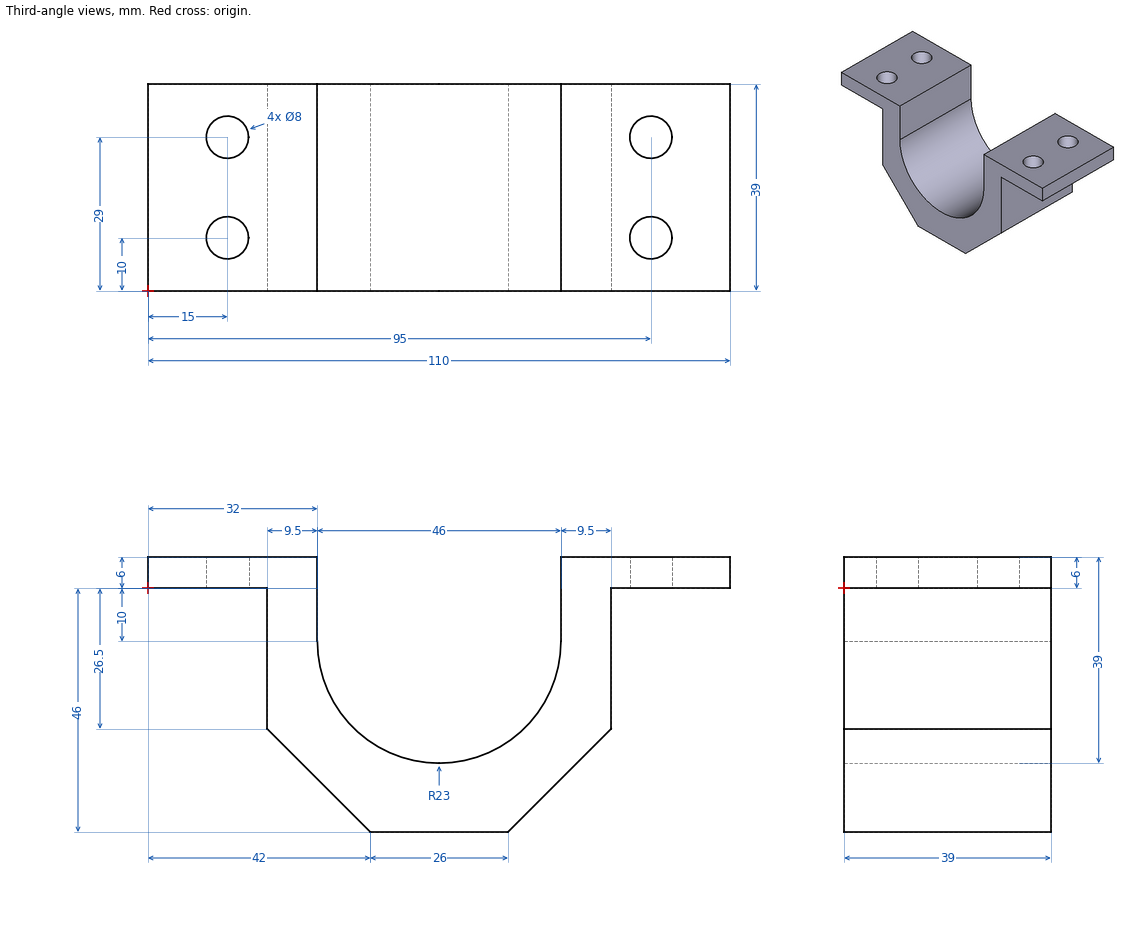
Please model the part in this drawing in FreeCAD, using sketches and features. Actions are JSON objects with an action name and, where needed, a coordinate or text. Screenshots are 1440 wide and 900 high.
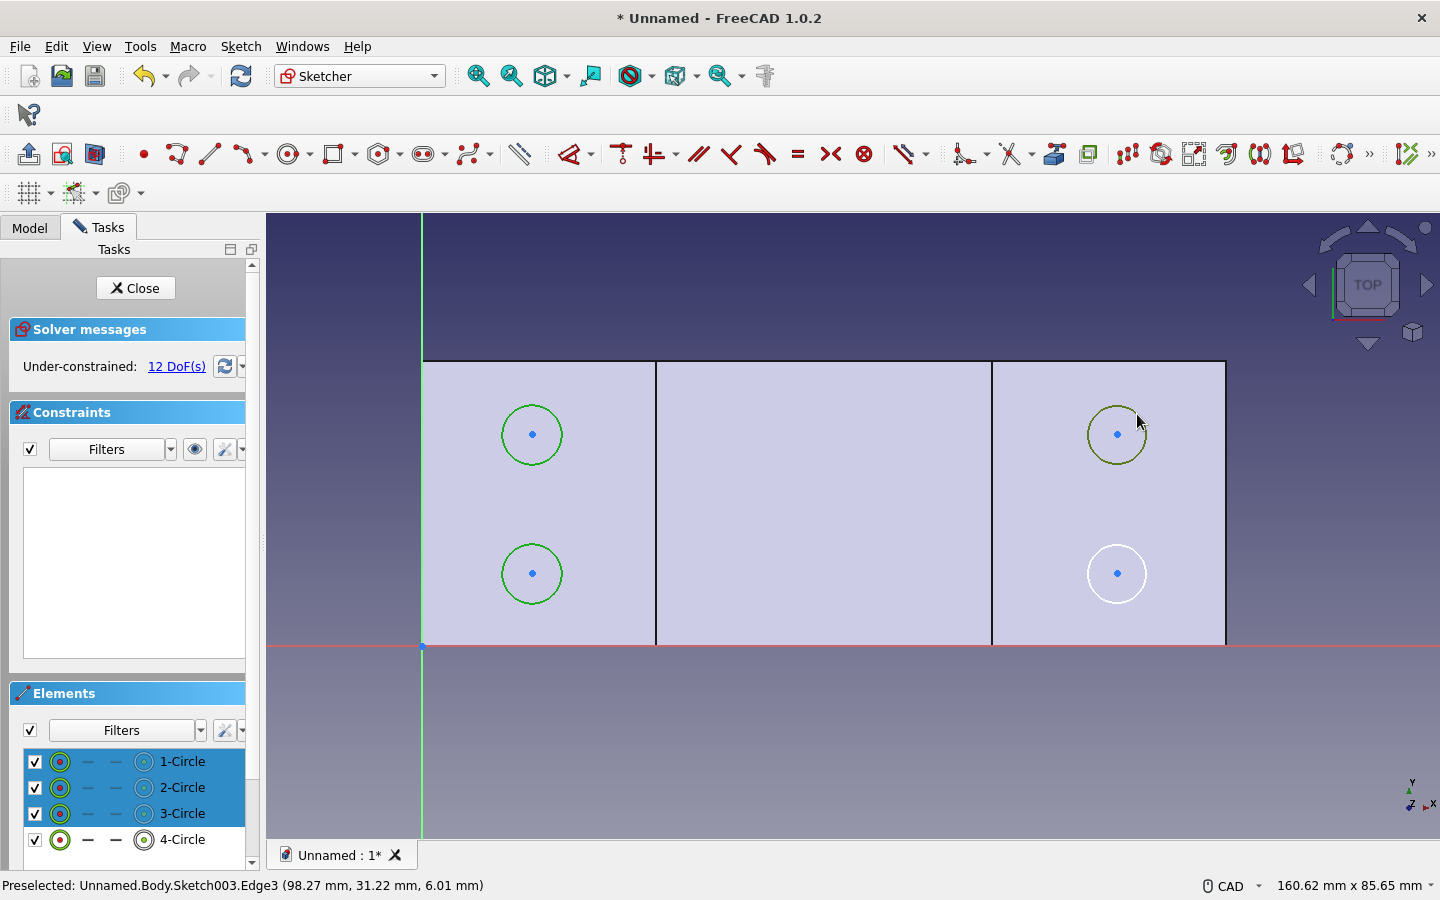
{"action": "left_click", "coordinate": [1137, 553]}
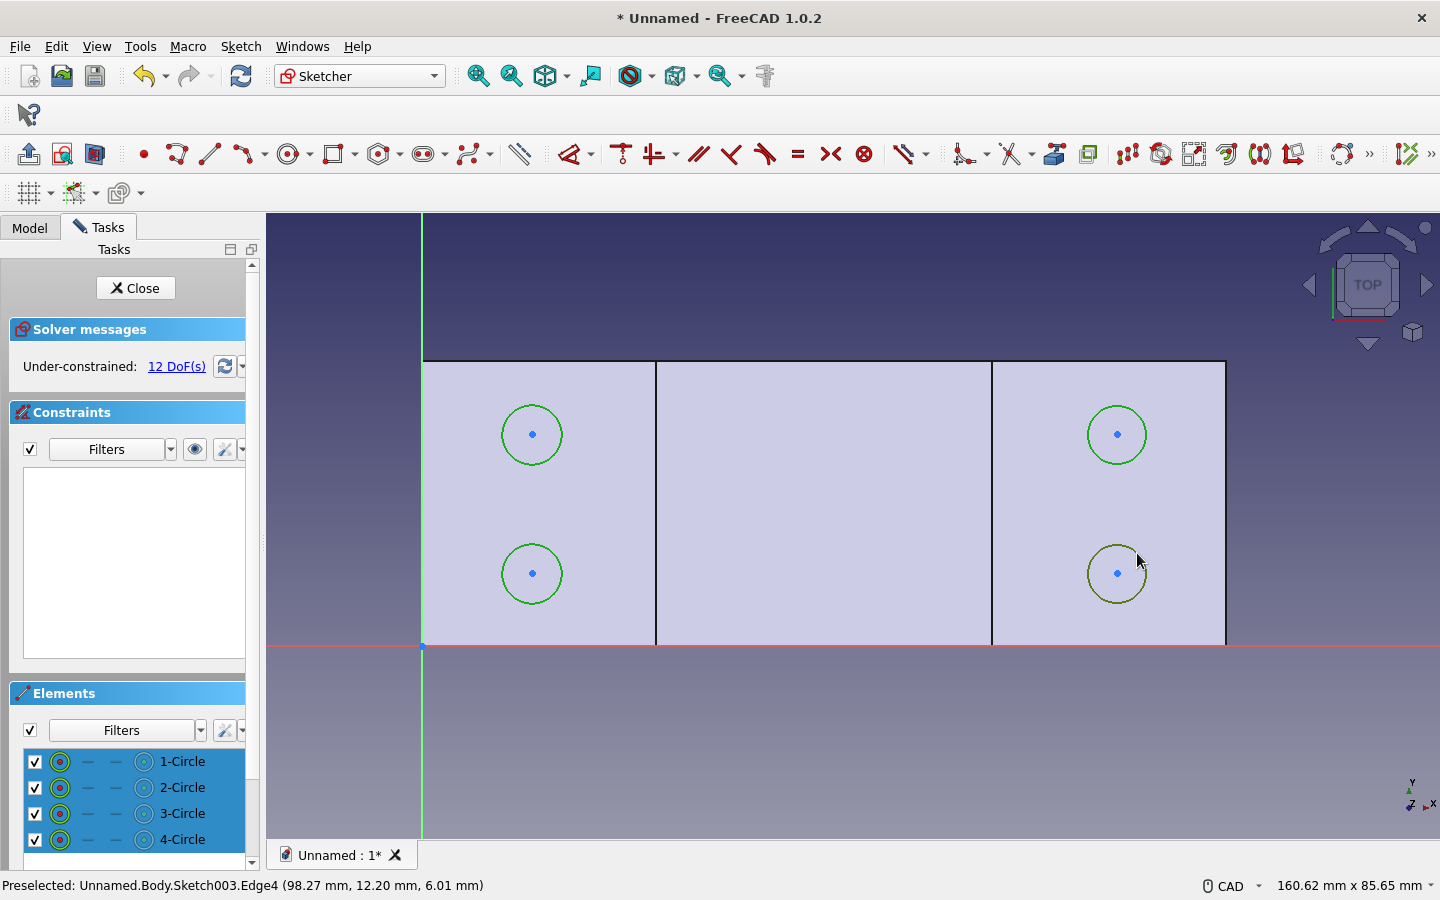
{"action": "key", "text": "e"}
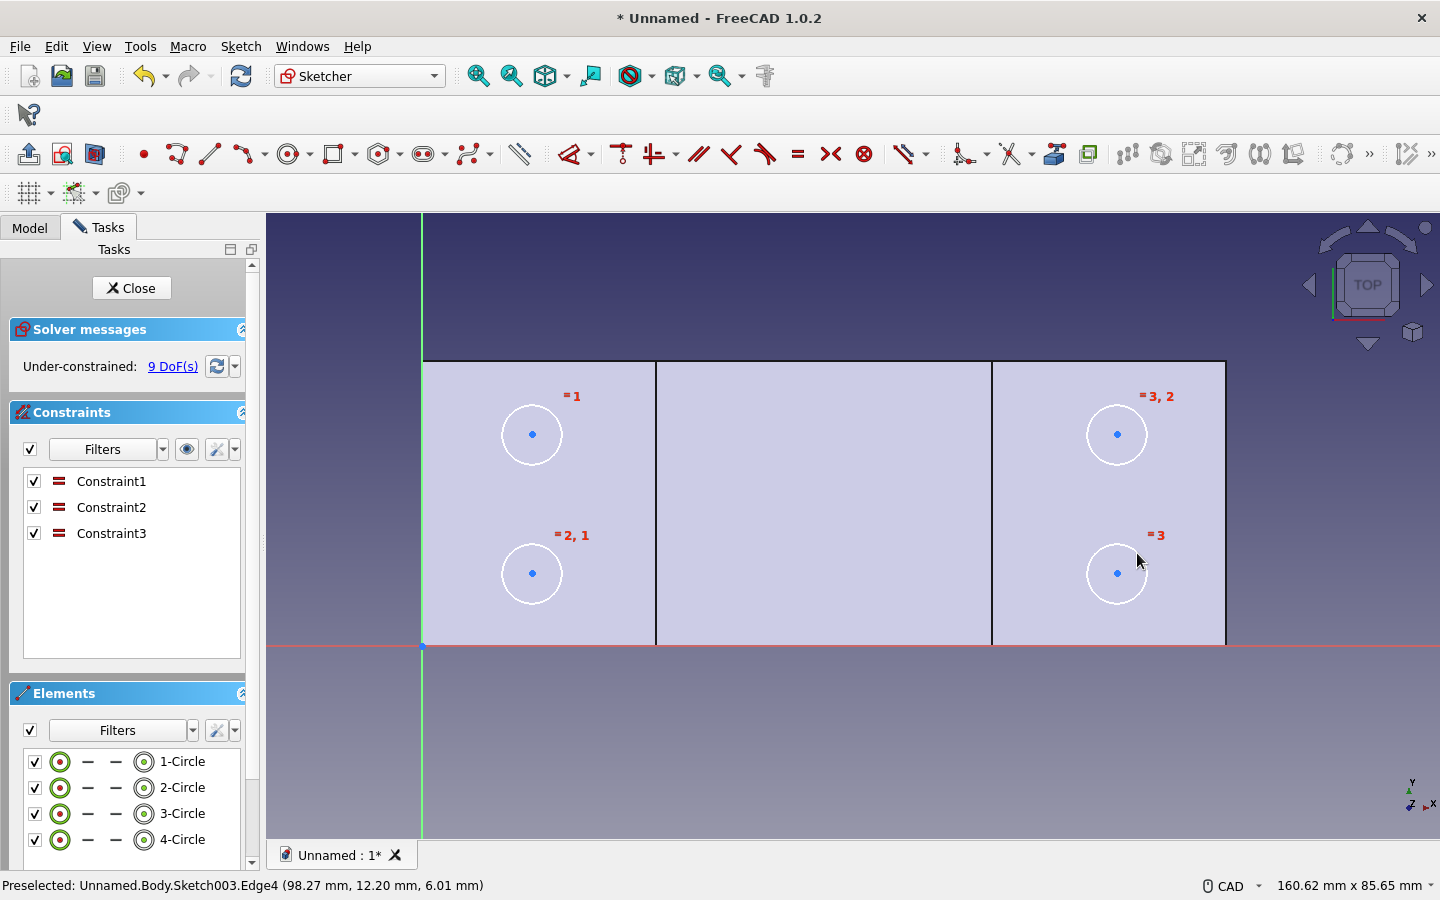
{"action": "left_click", "coordinate": [532, 435]}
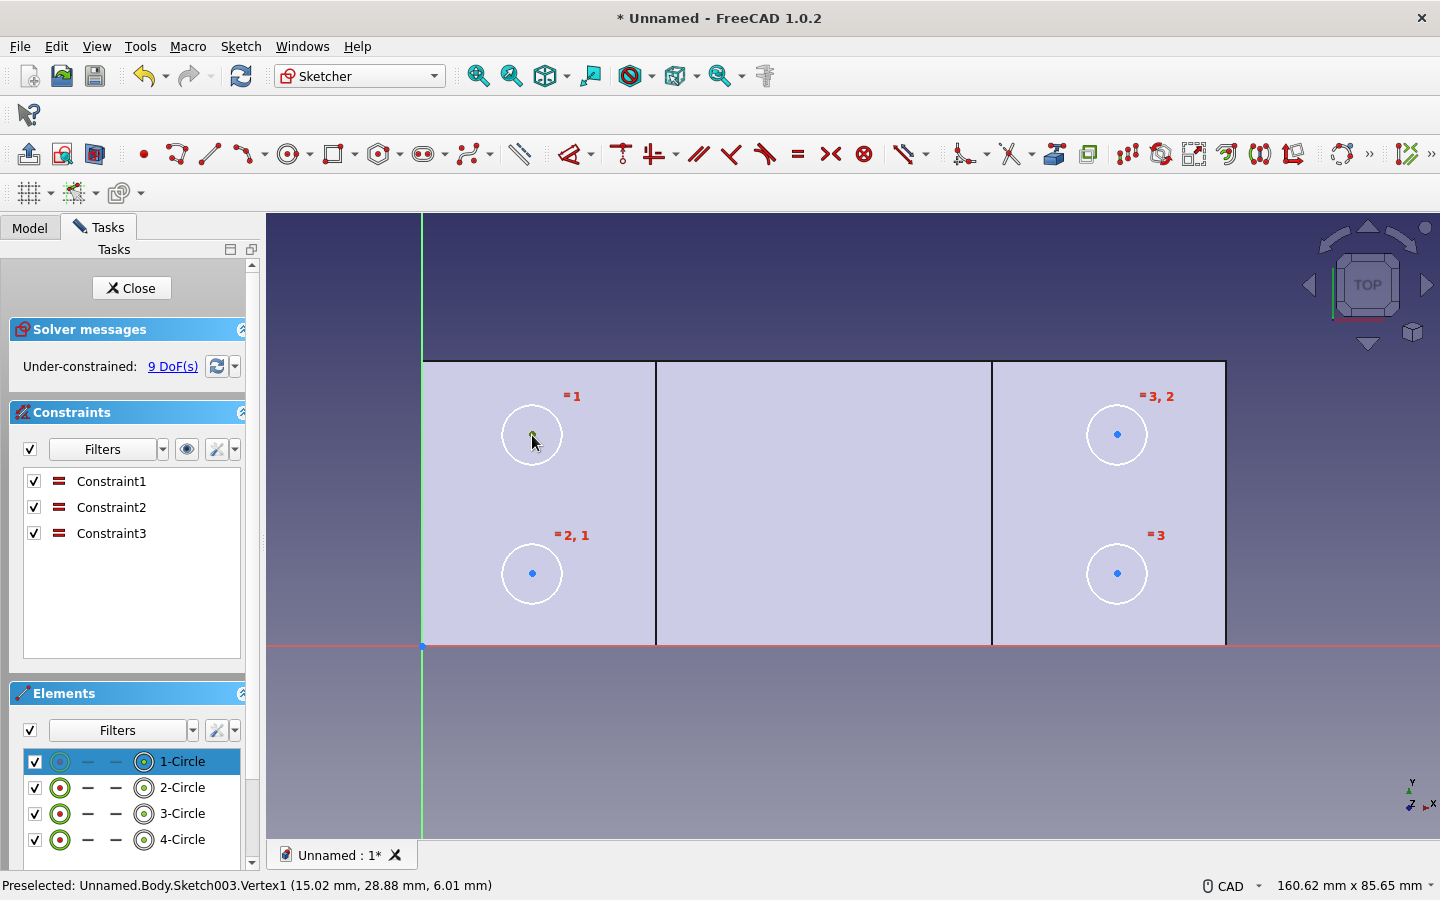
{"action": "left_click", "coordinate": [532, 574]}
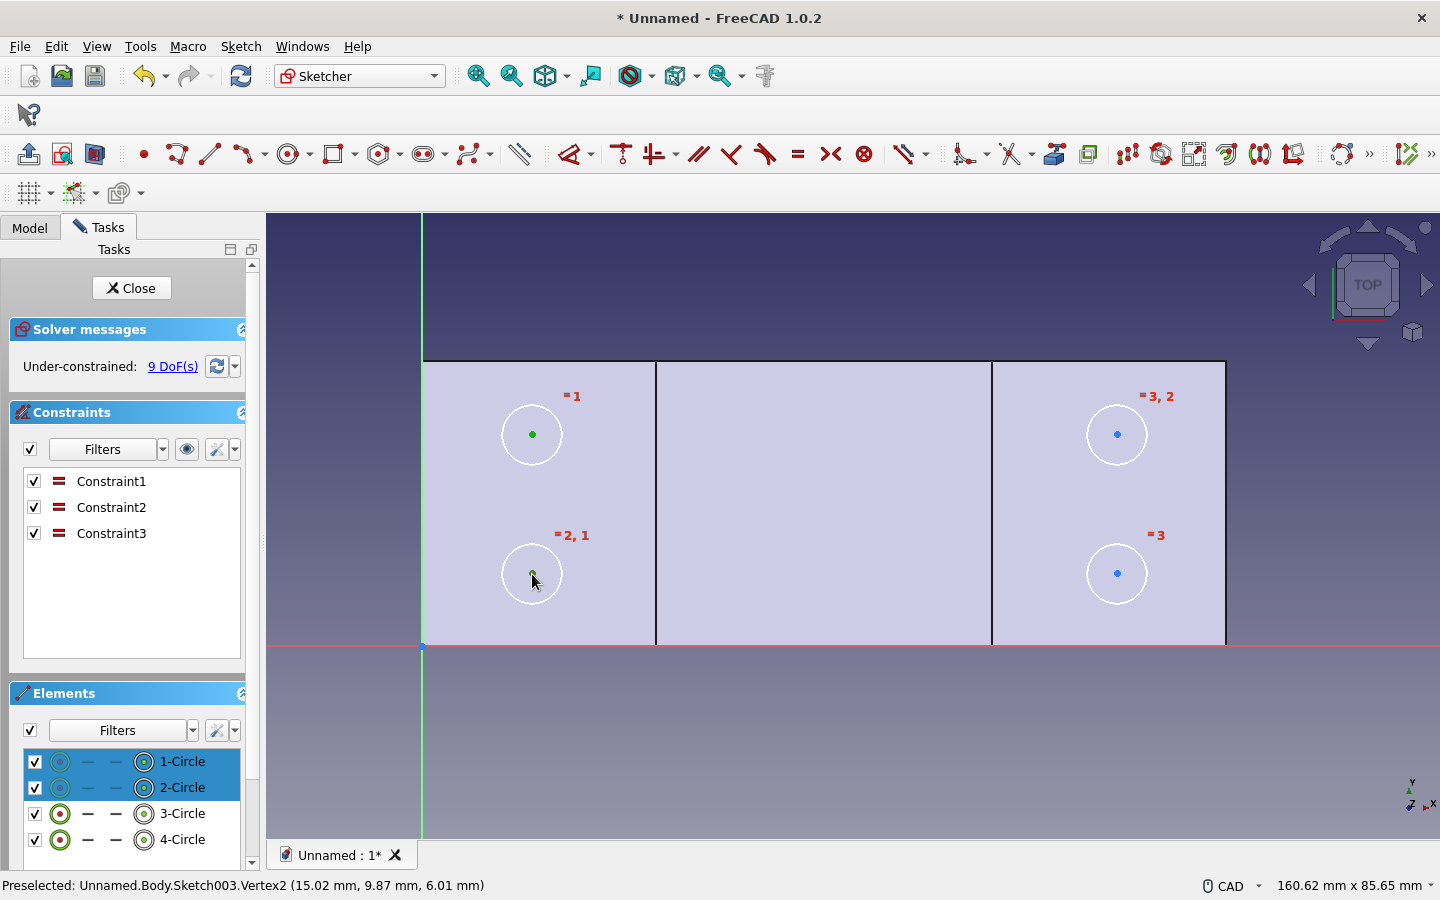
{"action": "key", "text": "v"}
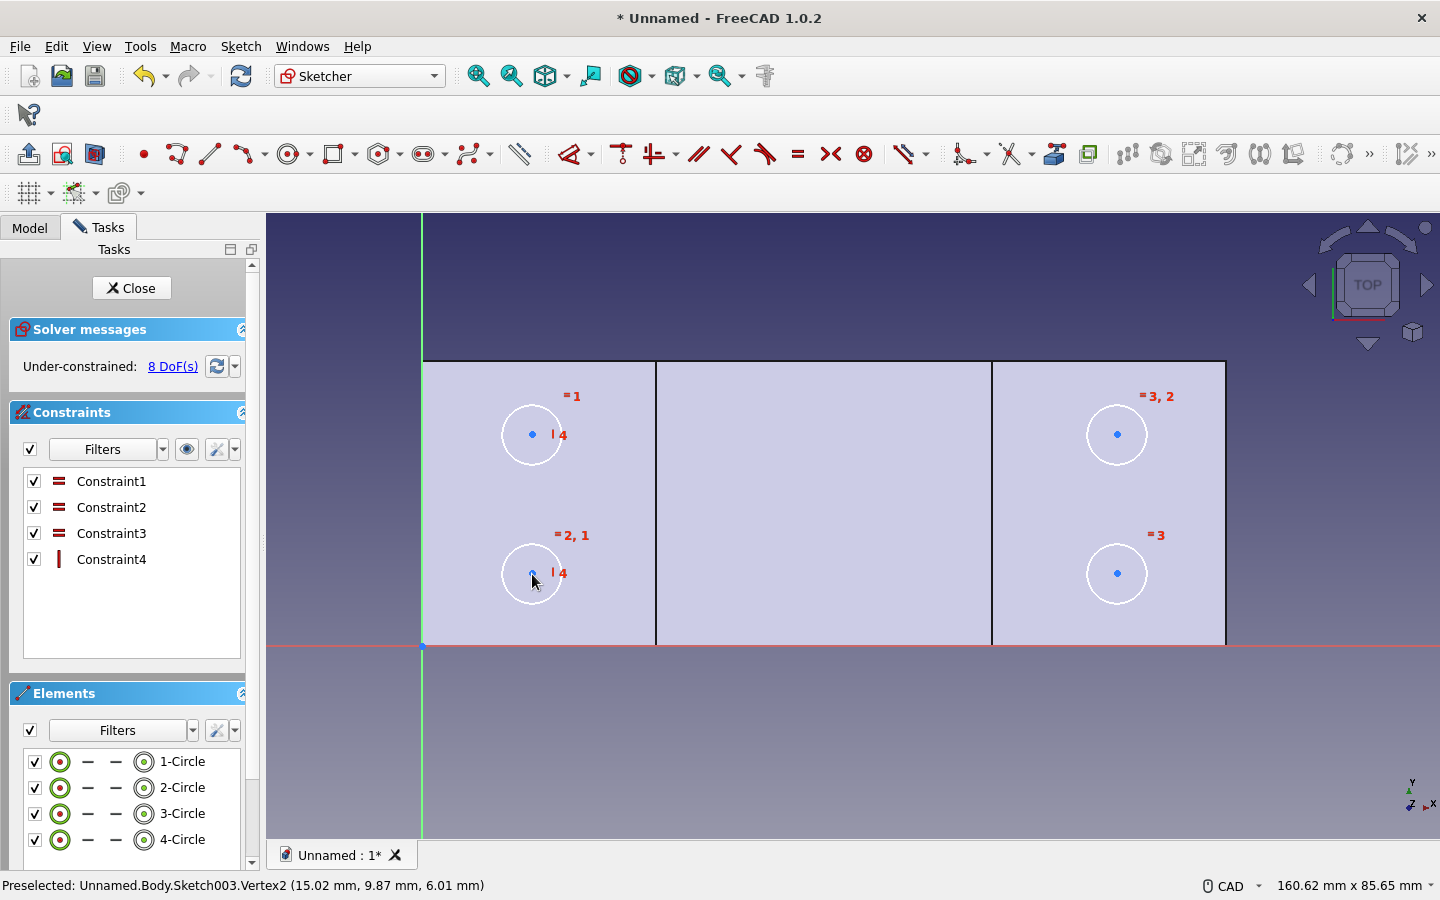
{"action": "left_click", "coordinate": [532, 435]}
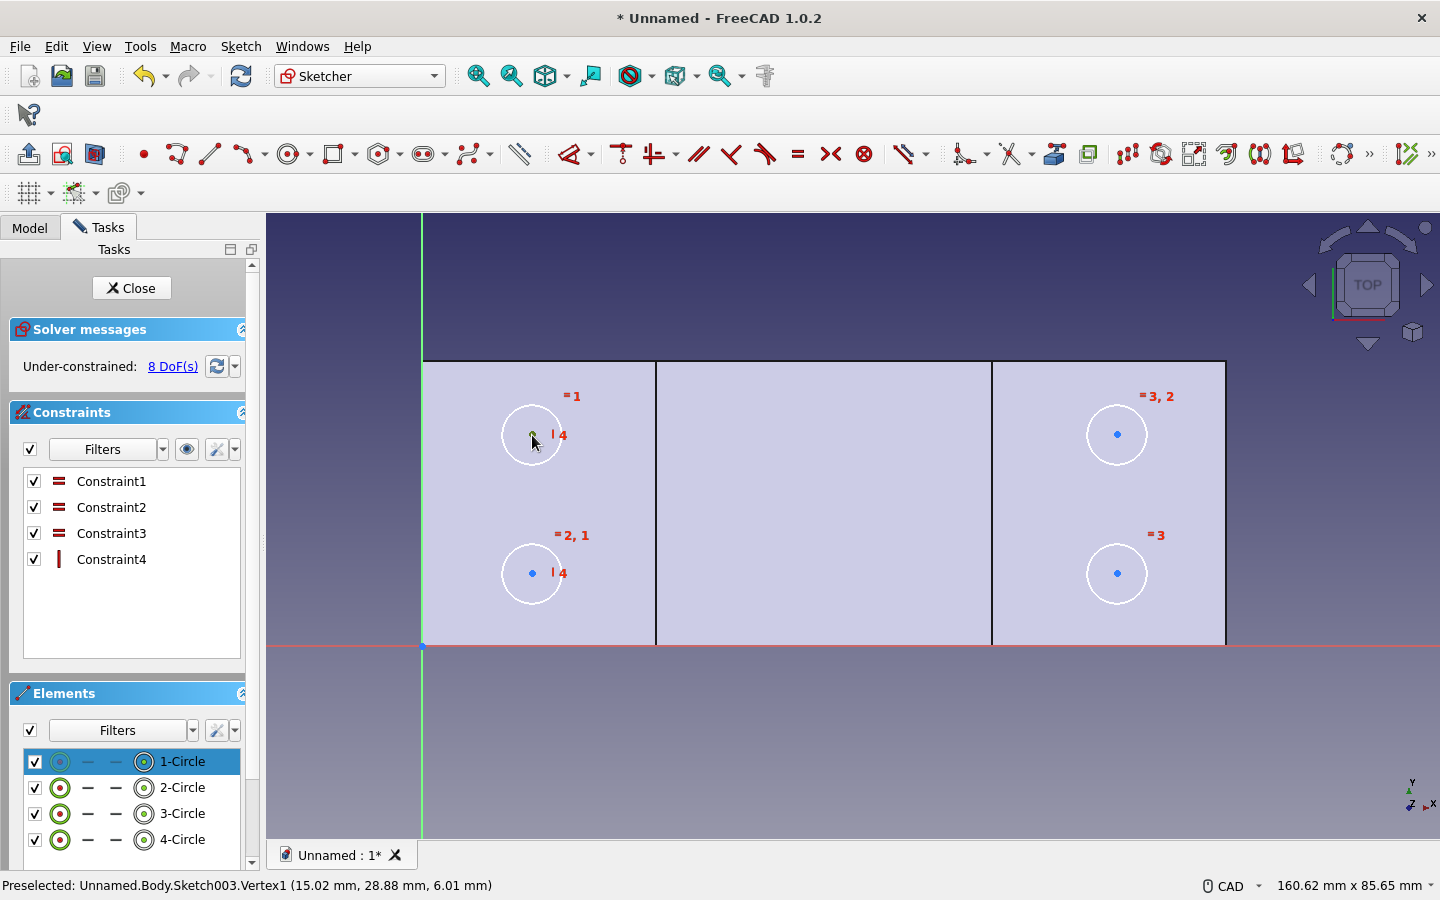
{"action": "left_click", "coordinate": [1117, 435]}